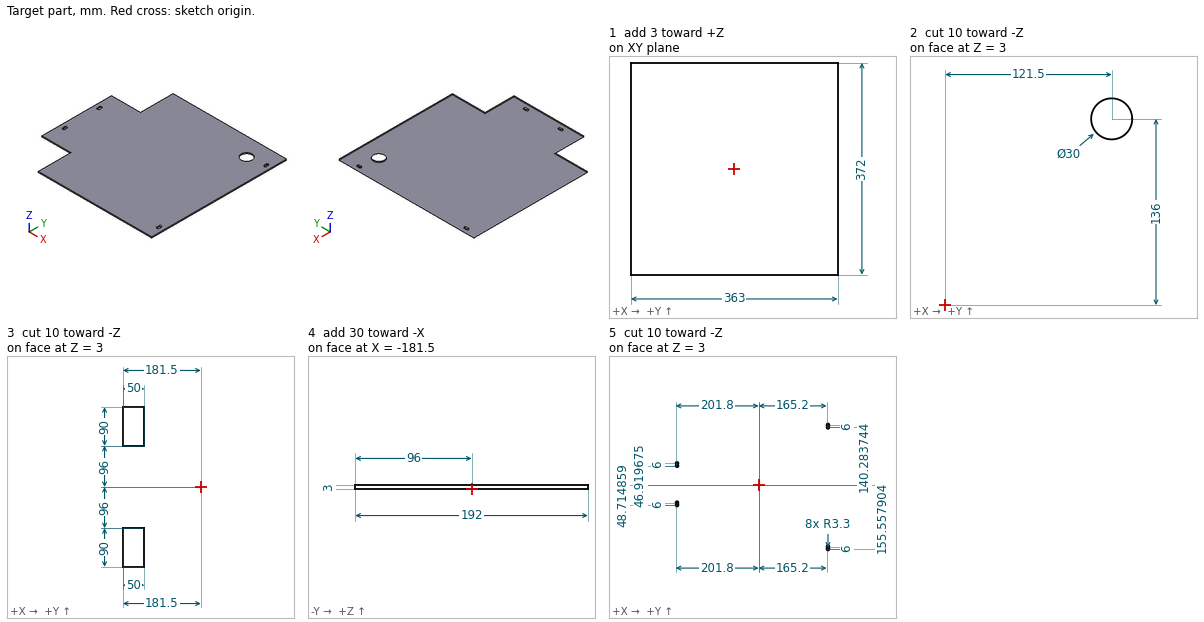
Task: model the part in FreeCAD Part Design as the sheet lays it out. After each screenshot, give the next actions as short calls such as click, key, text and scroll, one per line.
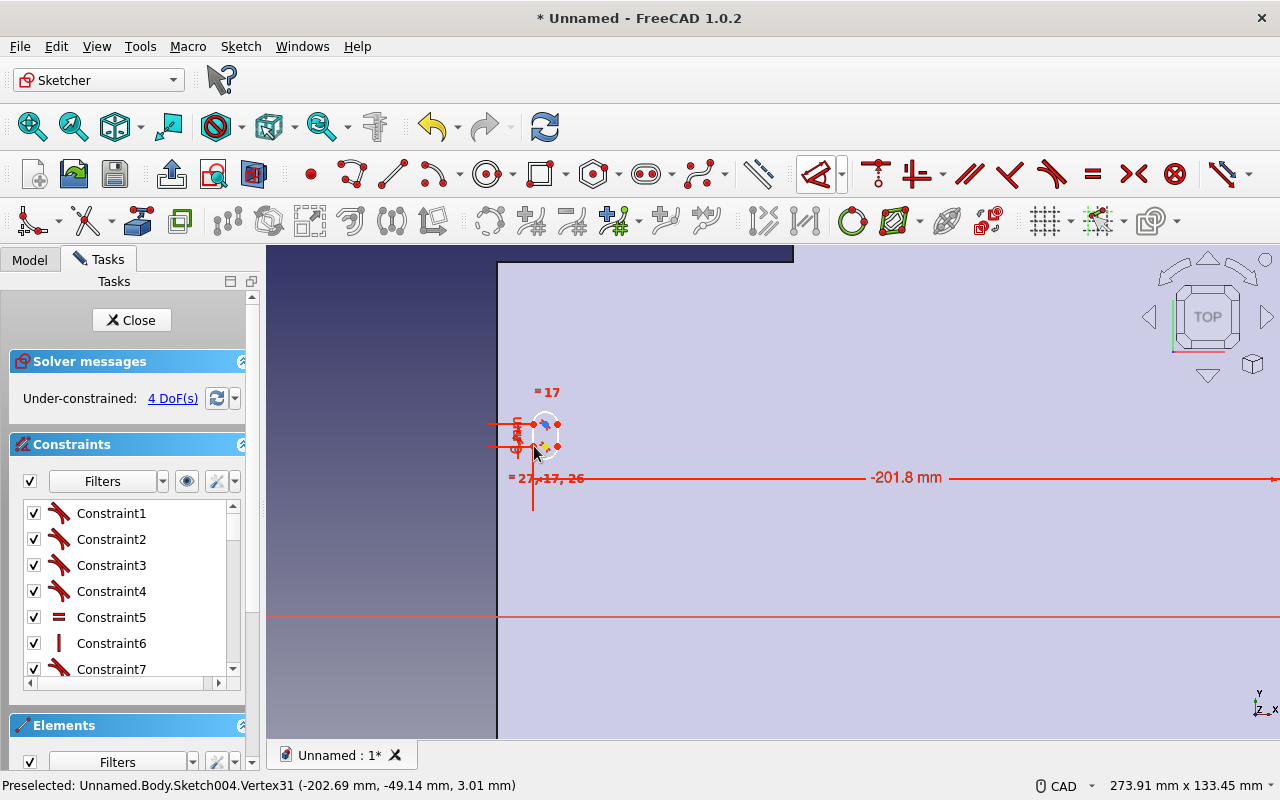
click(533, 447)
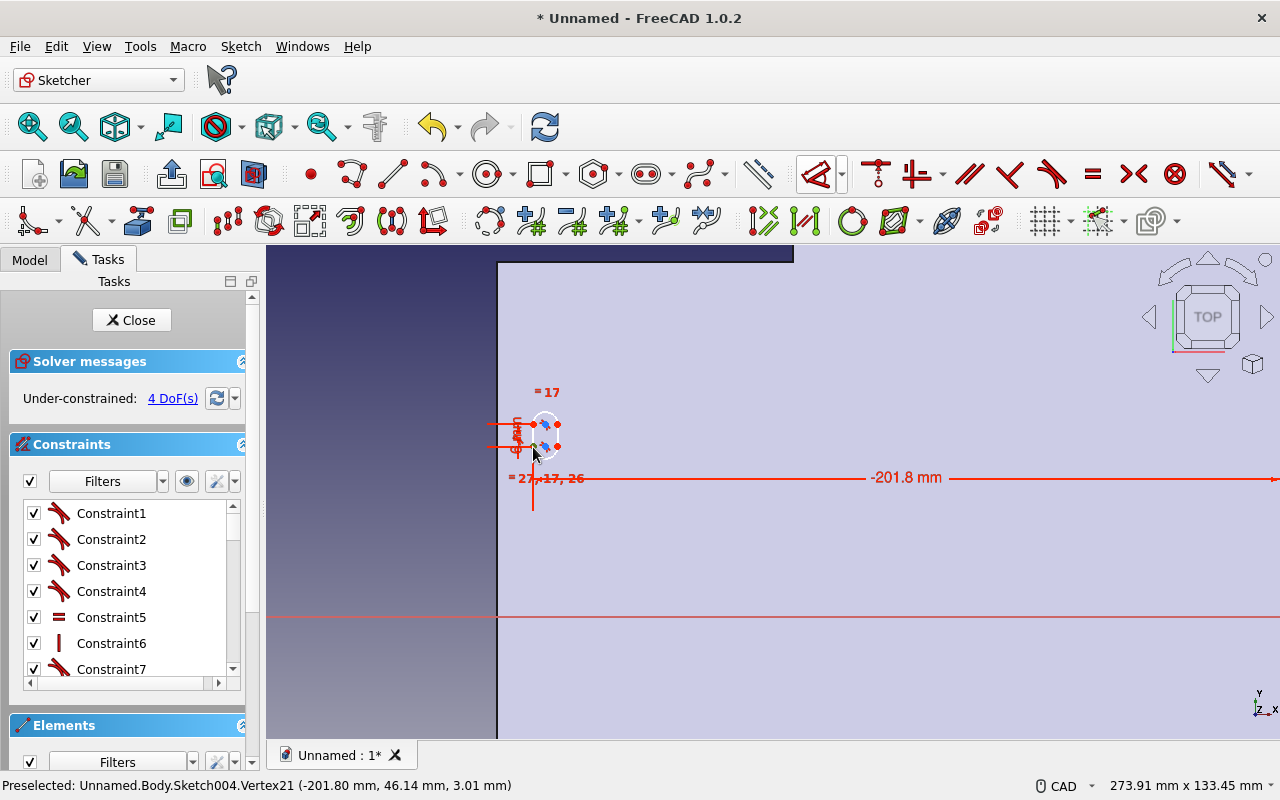
key(i)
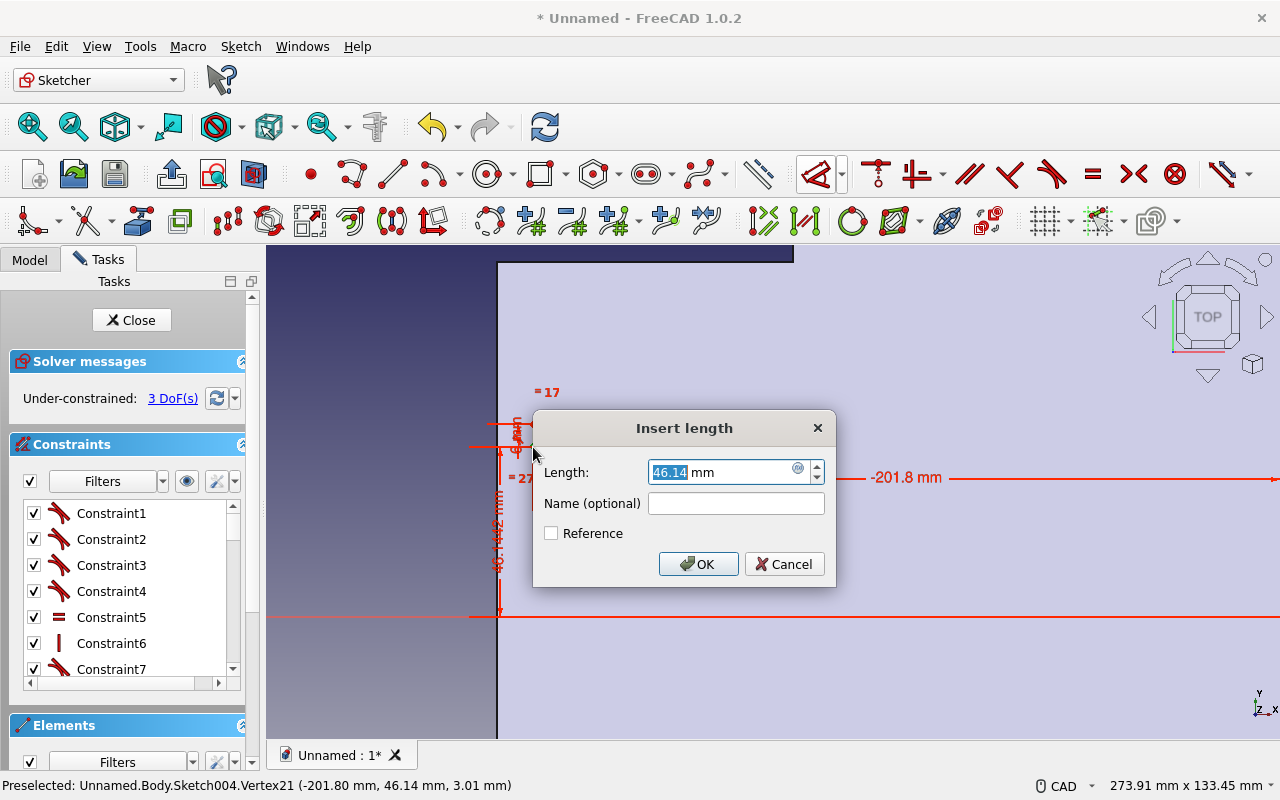
text(46.919675)
key(Return)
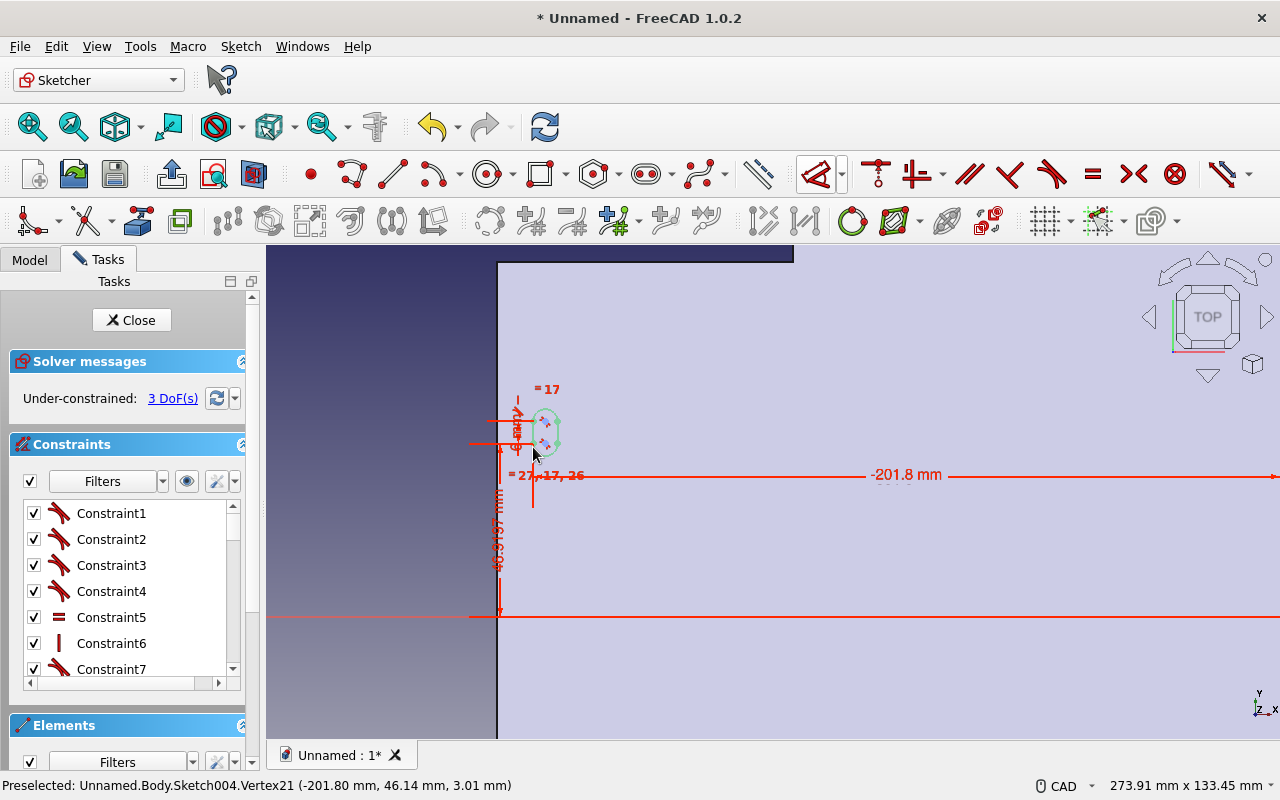
scroll(534, 445, down, 7)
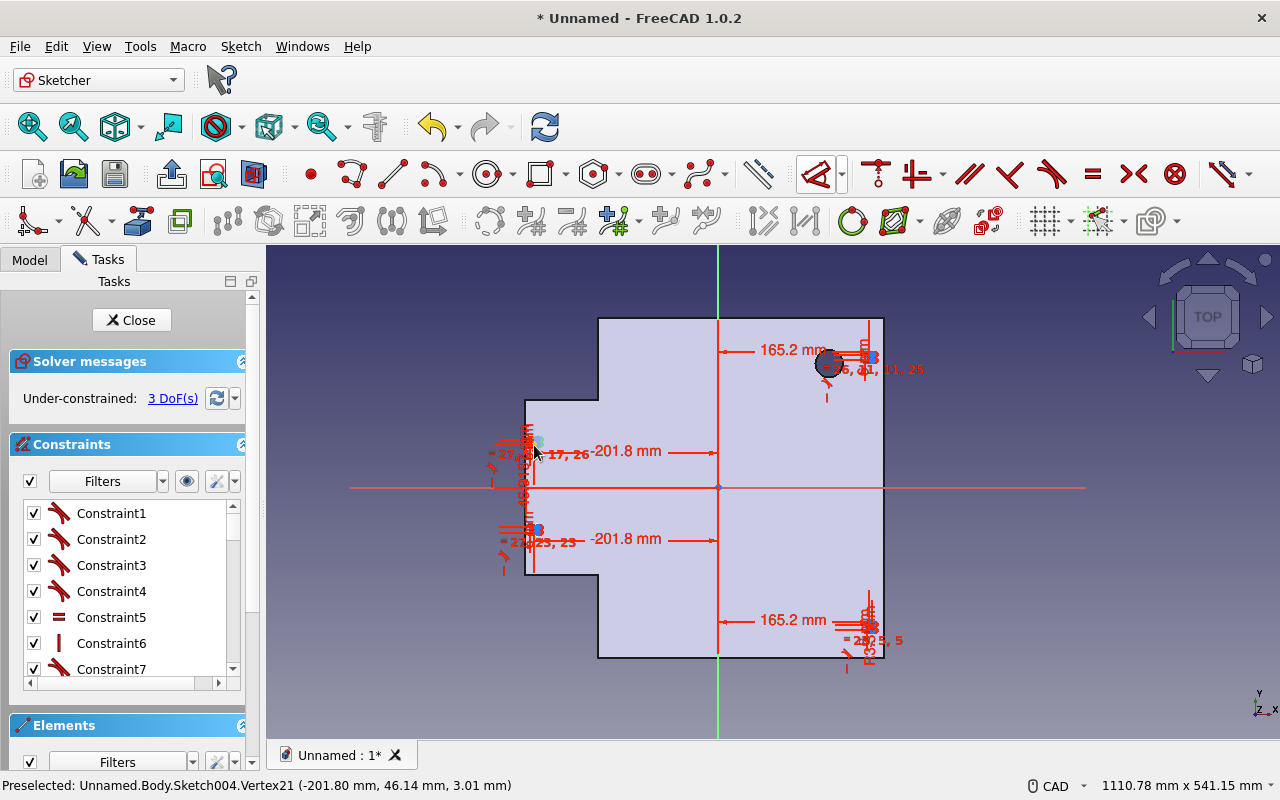
scroll(534, 533, up, 7)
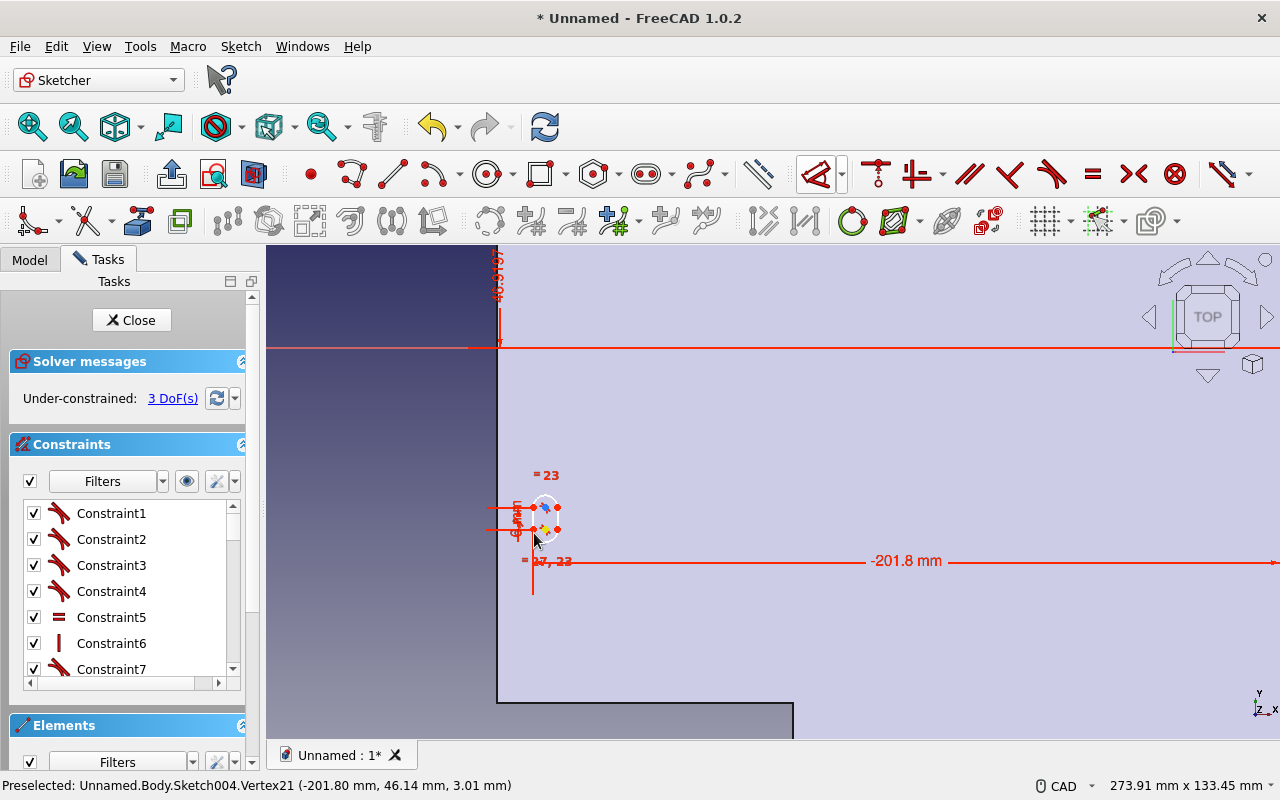
click(533, 530)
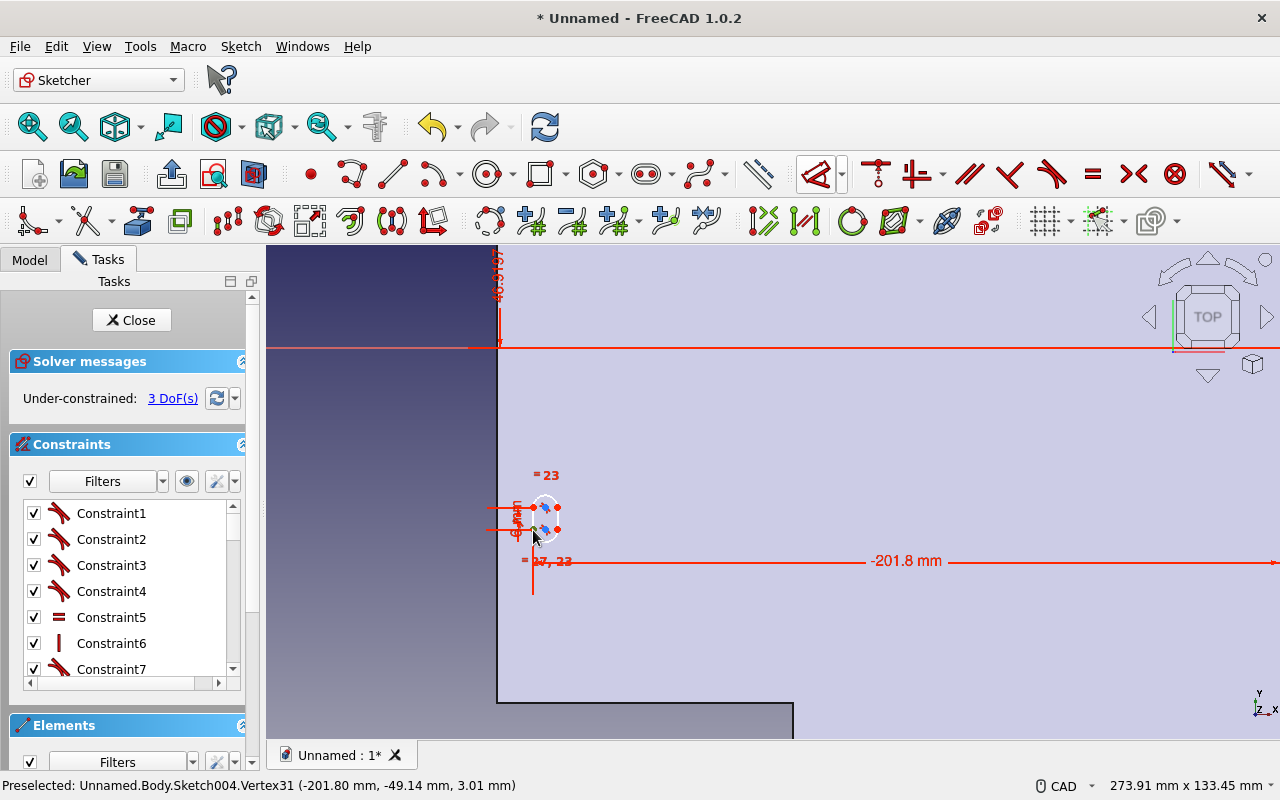
key(i)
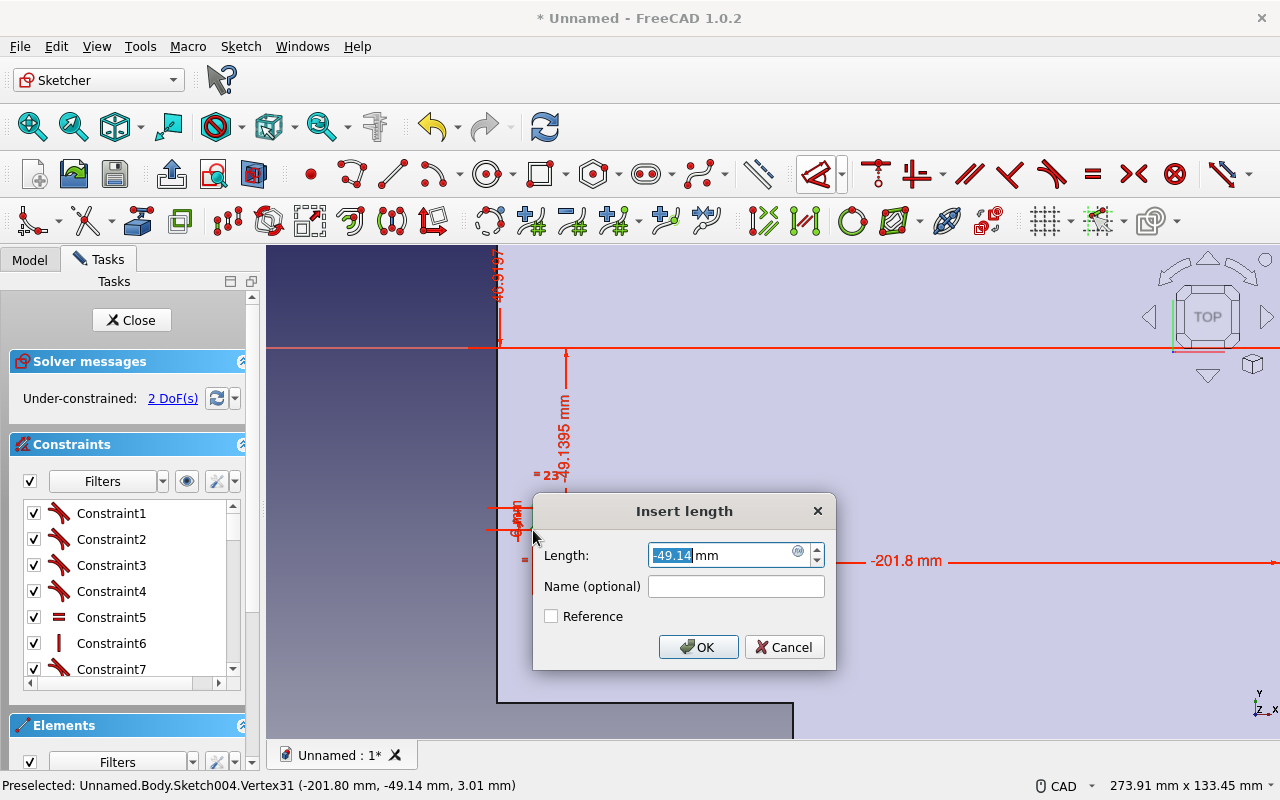
text(-48.714859)
key(Return)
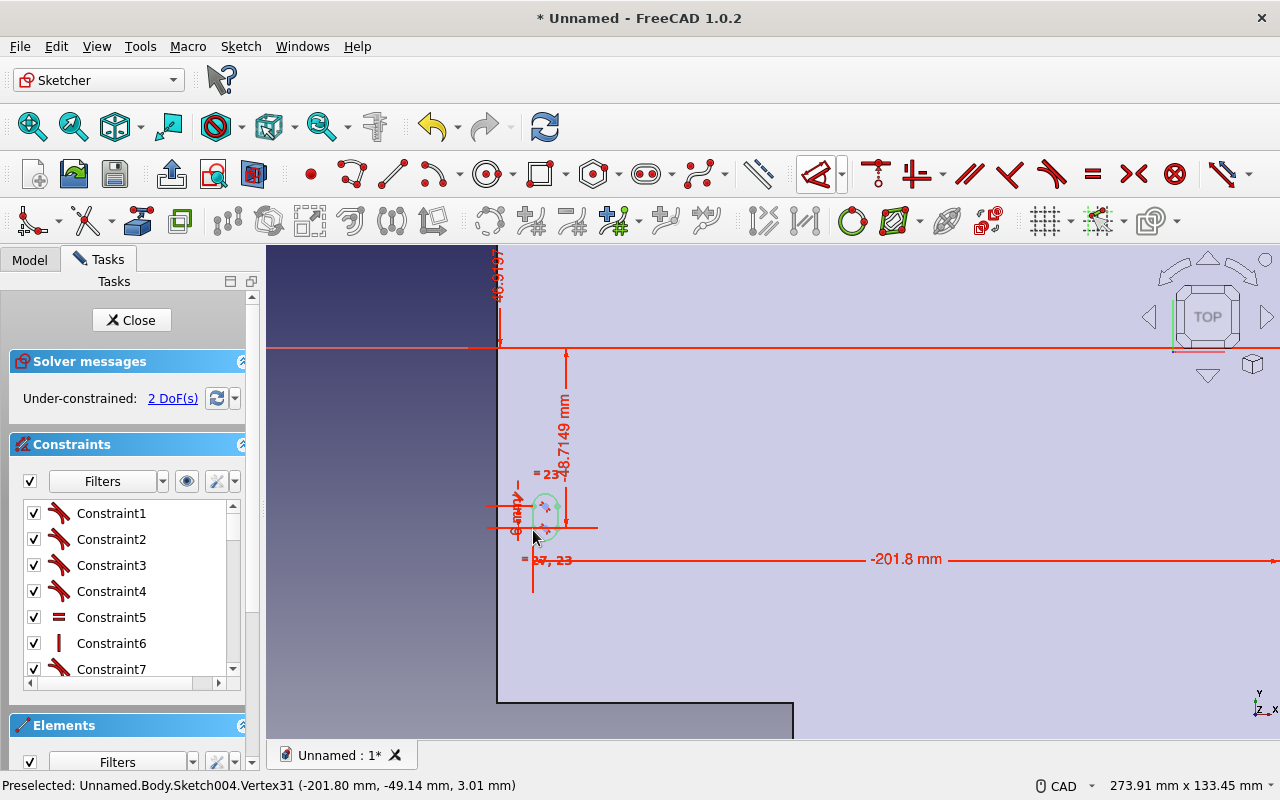
scroll(534, 534, down, 7)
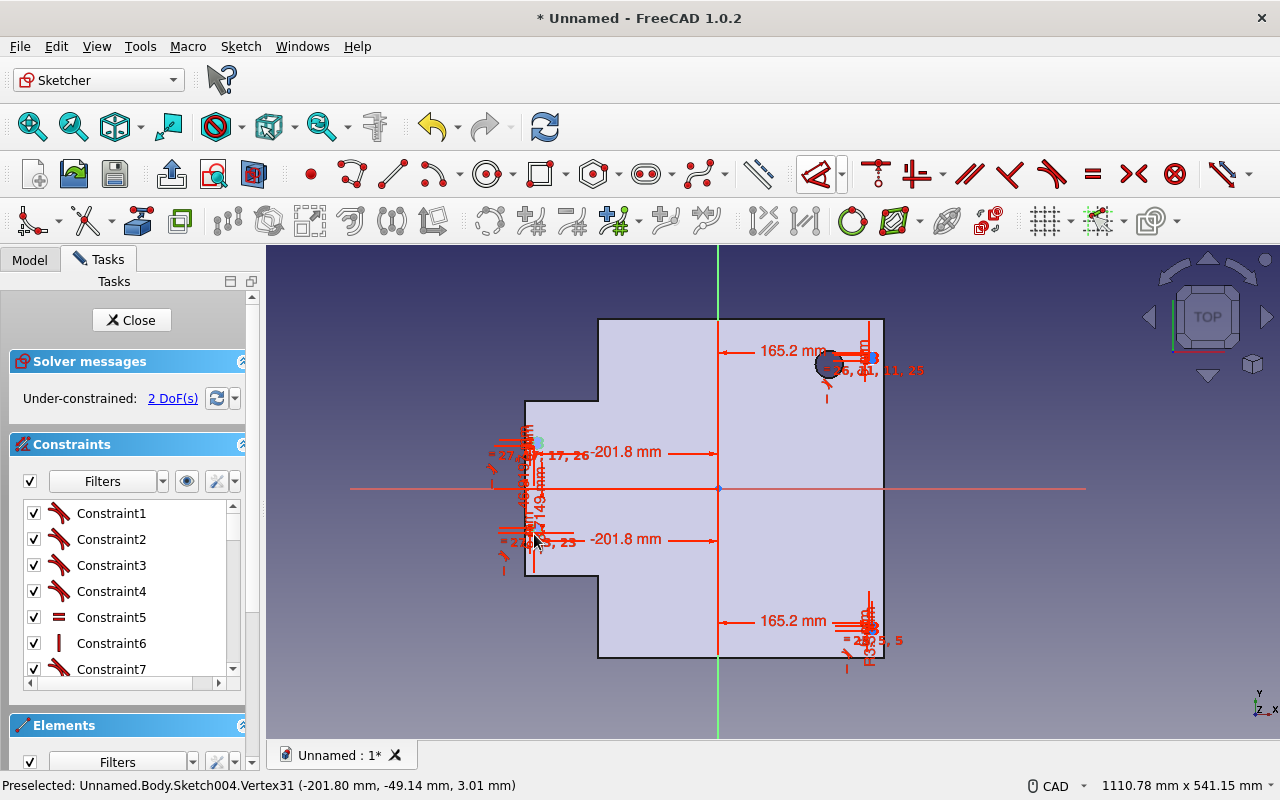
scroll(869, 631, up, 7)